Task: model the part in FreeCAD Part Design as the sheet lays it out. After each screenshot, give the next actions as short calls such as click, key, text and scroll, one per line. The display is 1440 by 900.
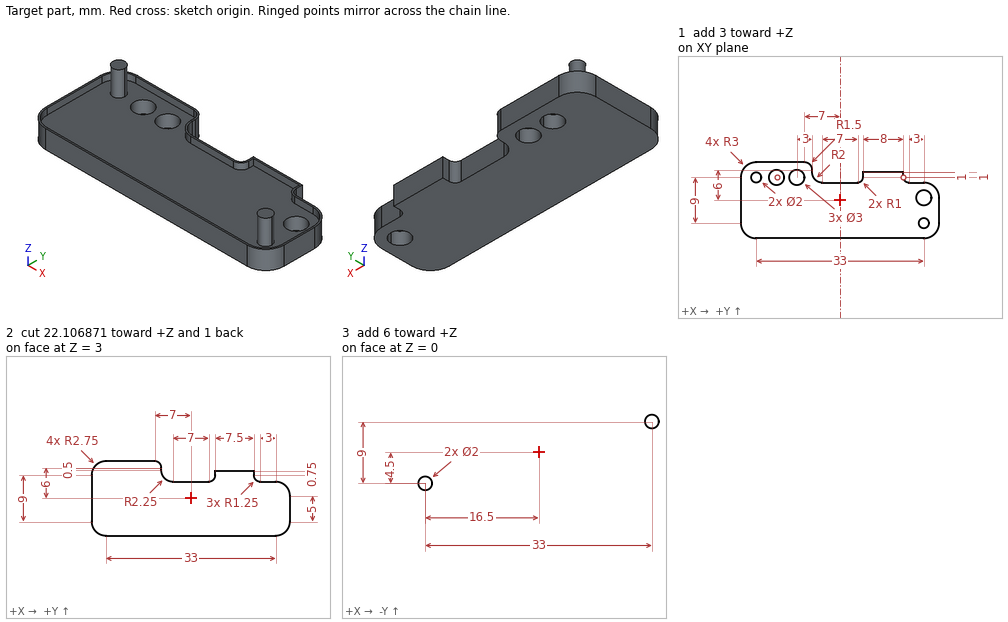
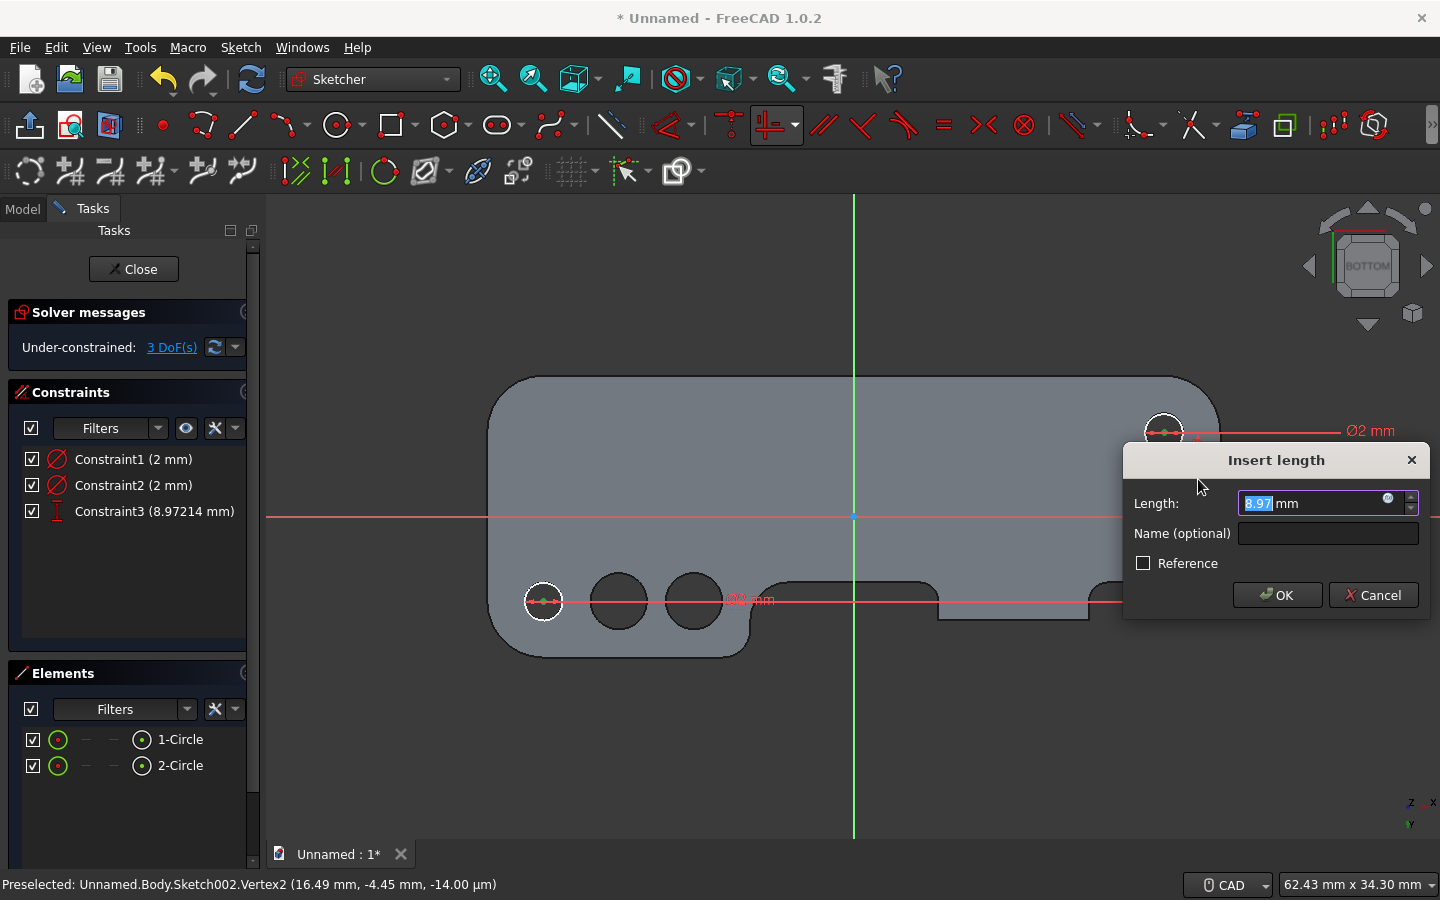
text(9)
key(Return)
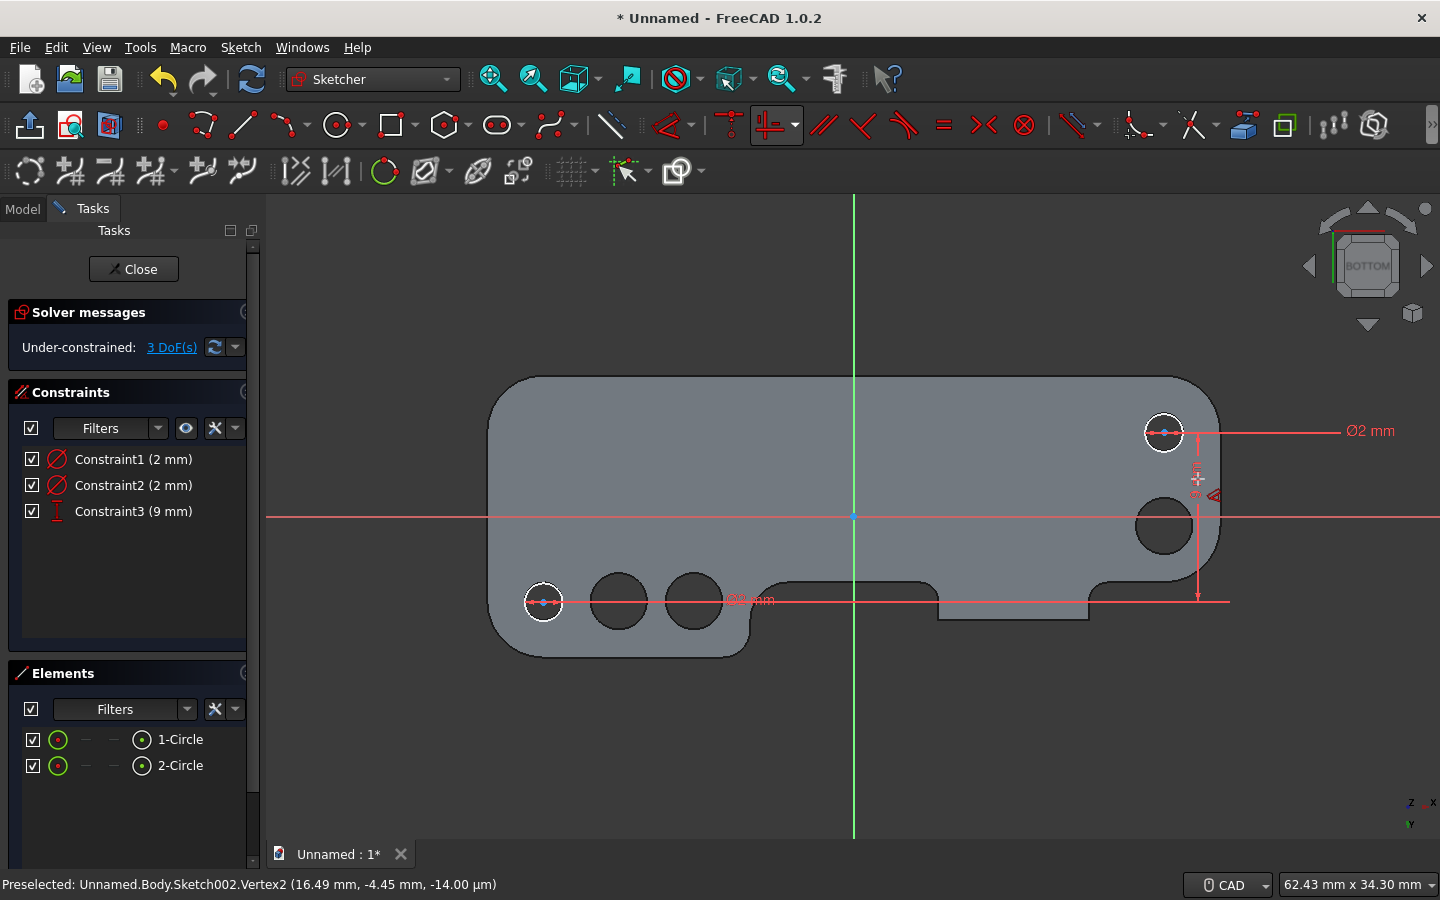
click(544, 602)
click(510, 559)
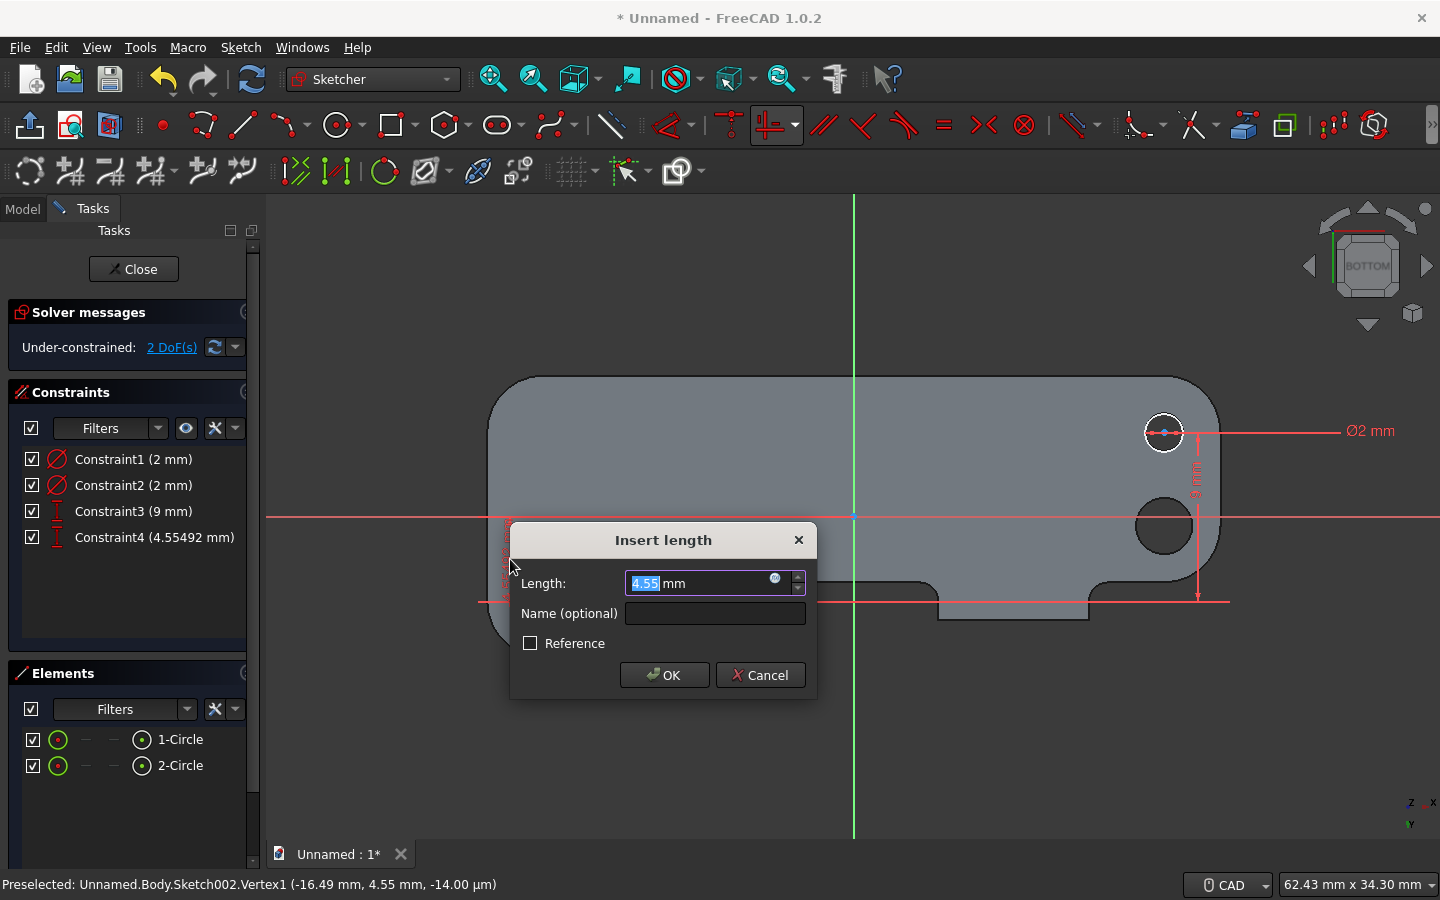
text(4.5)
key(Return)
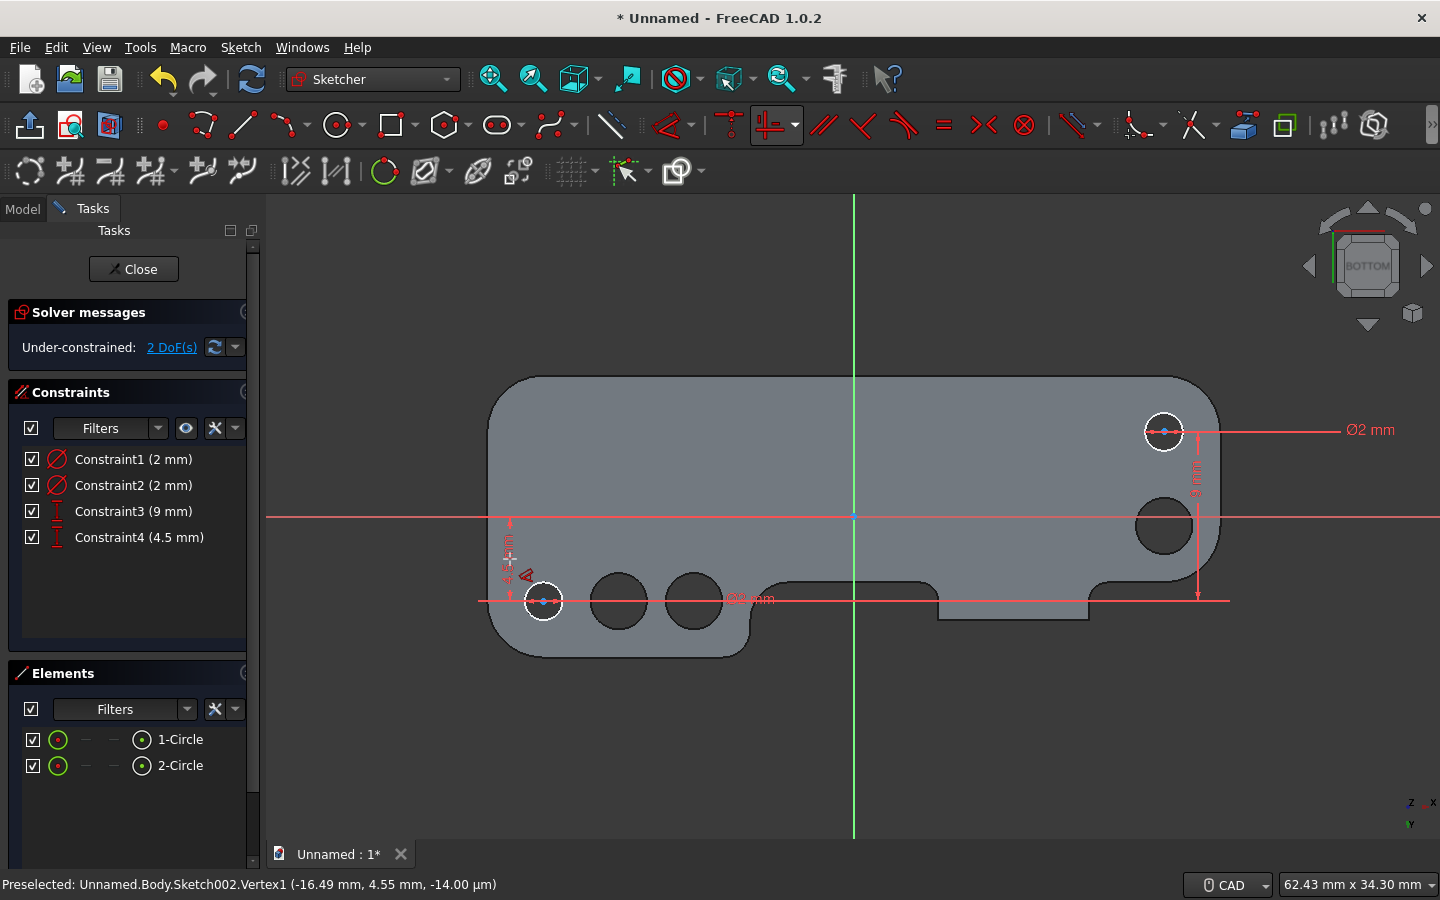
click(544, 601)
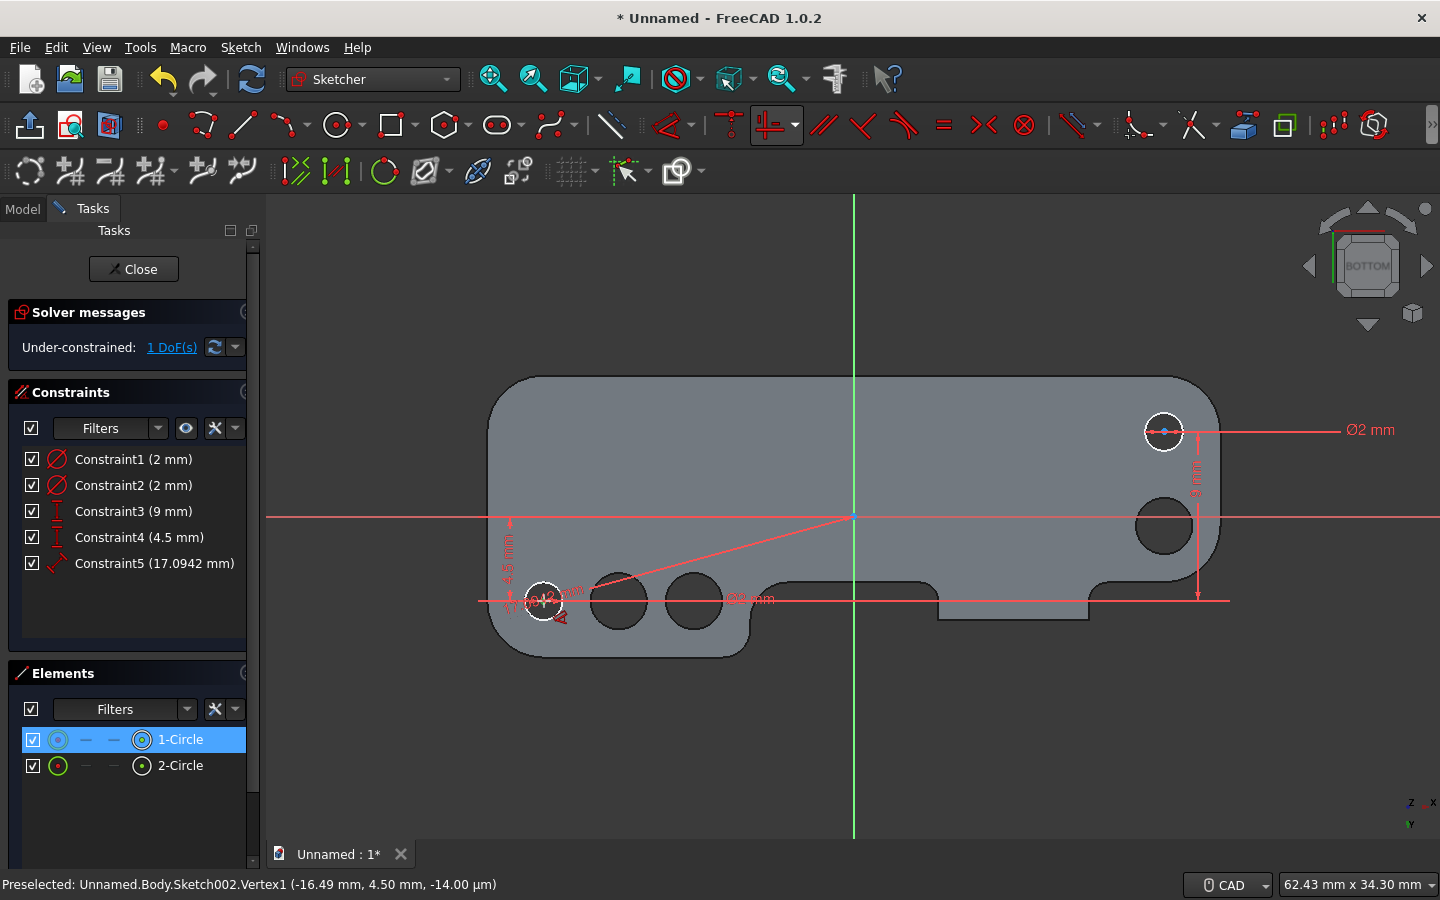
click(1164, 432)
click(711, 635)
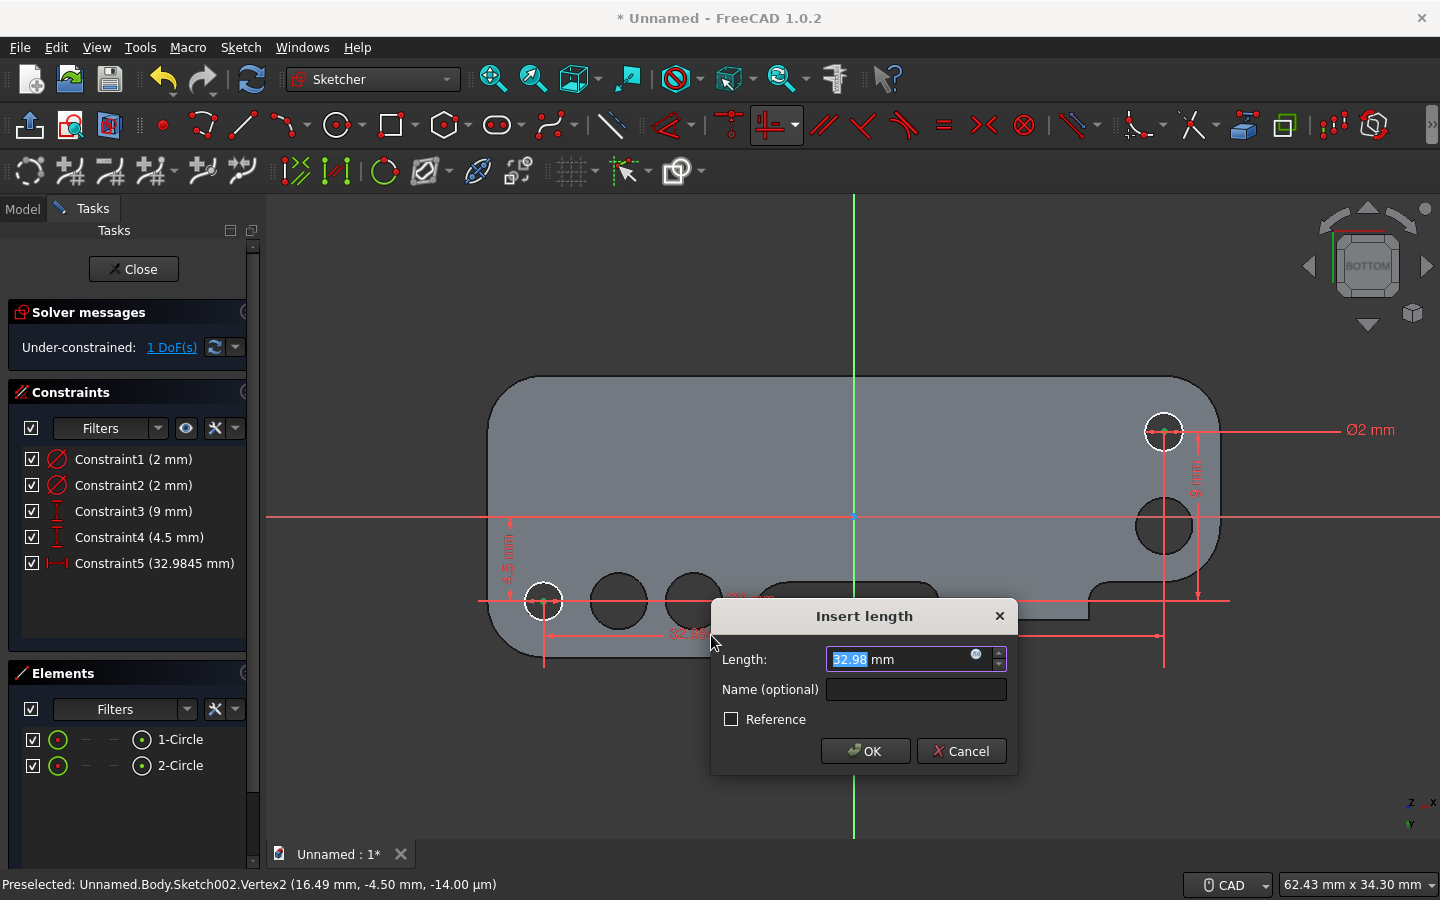
text(33)
key(Return)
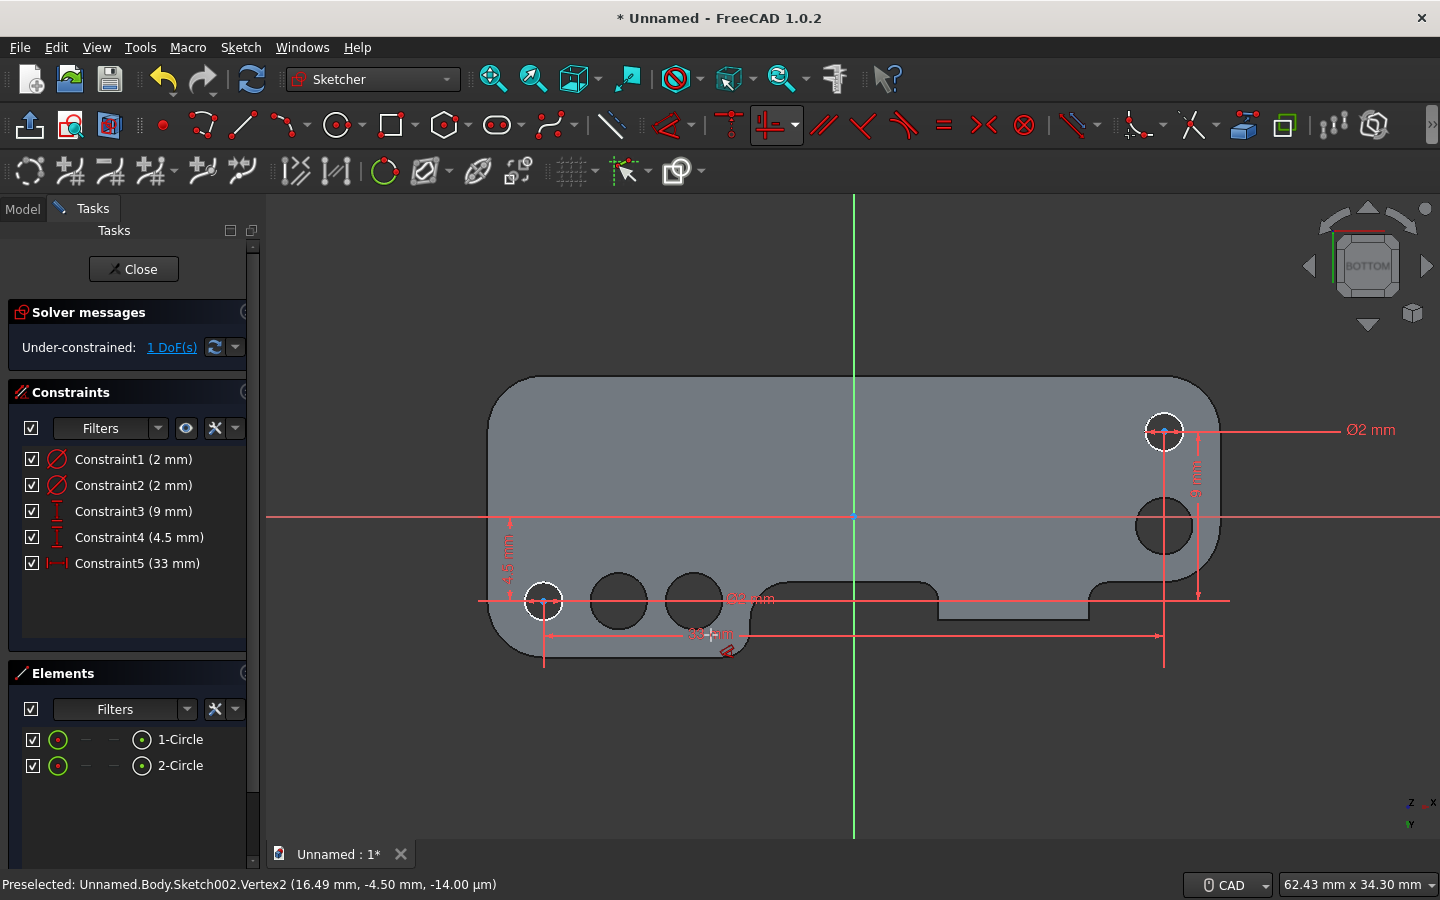
click(544, 601)
click(627, 635)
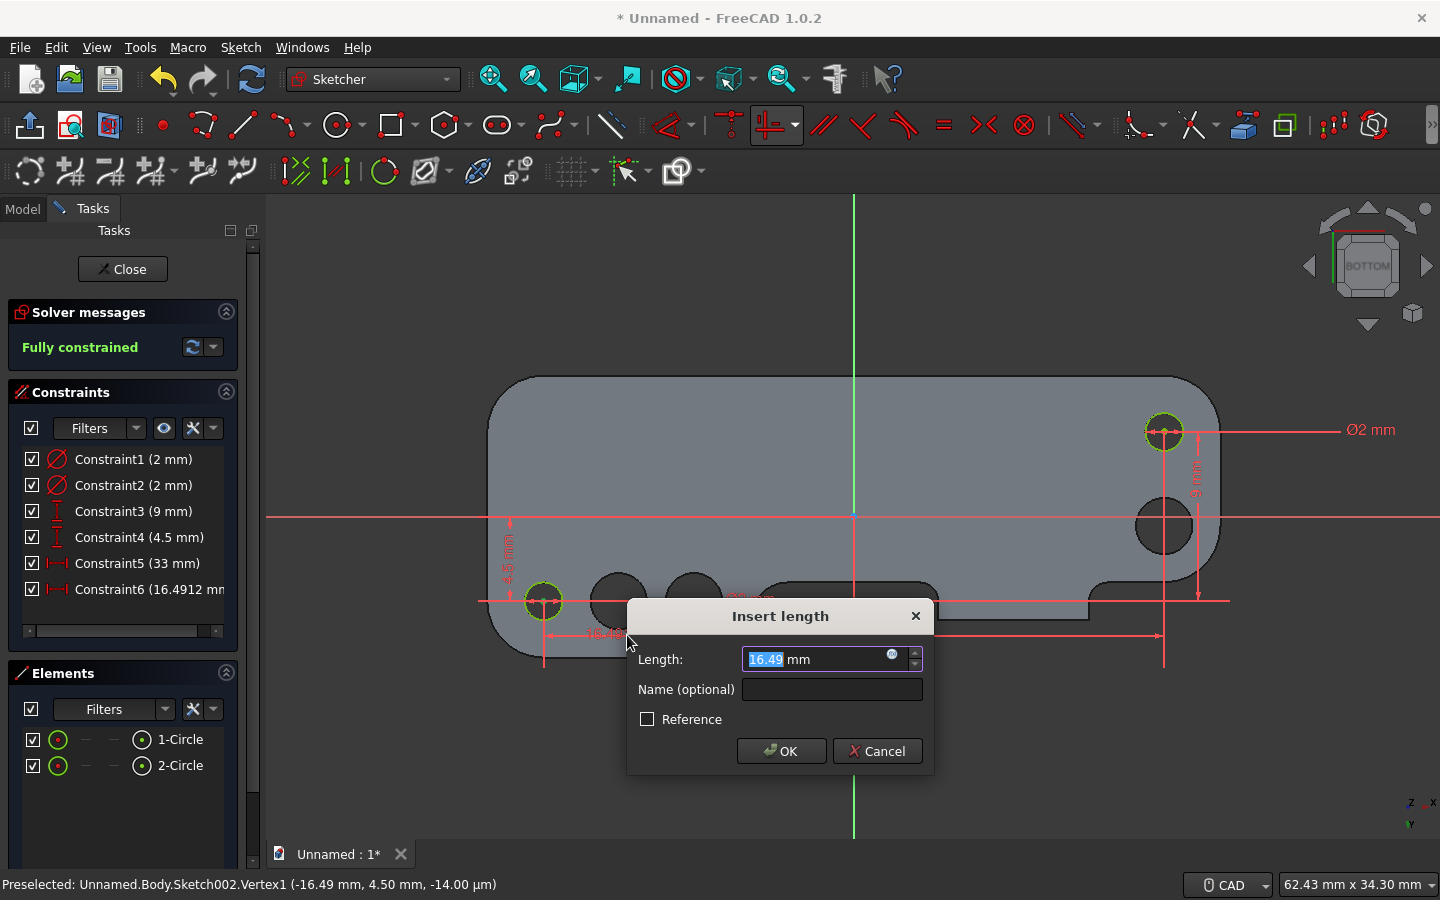
text(16.5)
key(Return)
key(Escape)